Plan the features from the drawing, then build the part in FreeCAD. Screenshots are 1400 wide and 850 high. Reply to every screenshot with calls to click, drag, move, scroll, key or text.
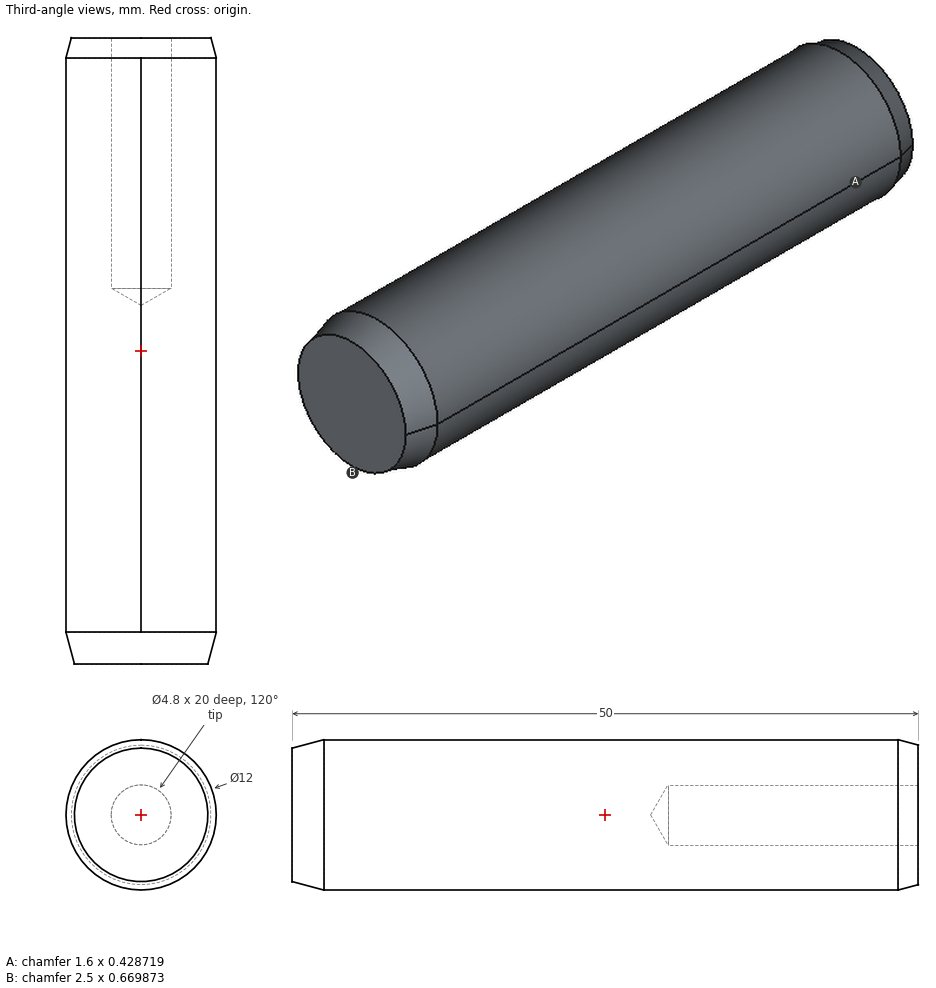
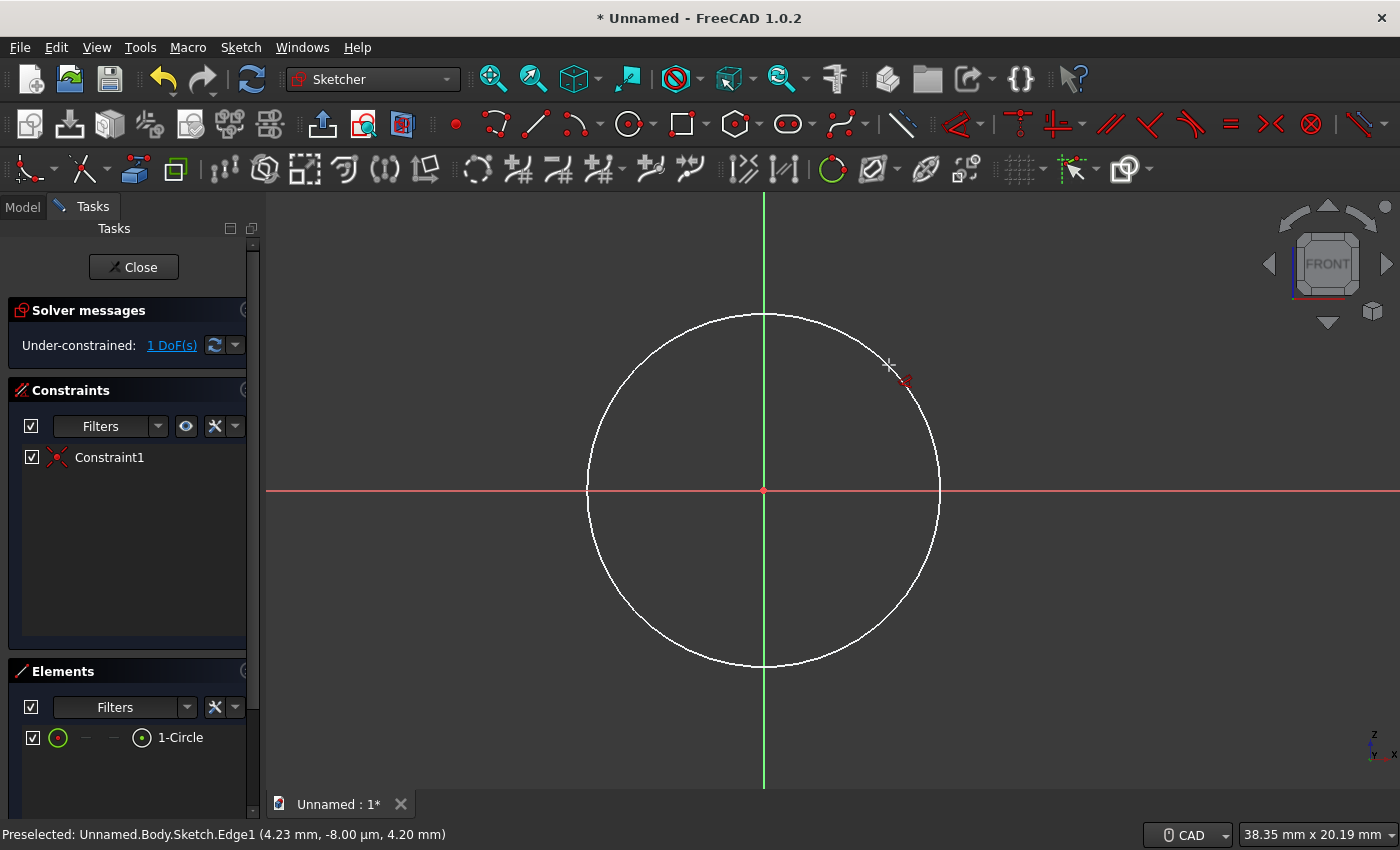
click(888, 365)
click(911, 342)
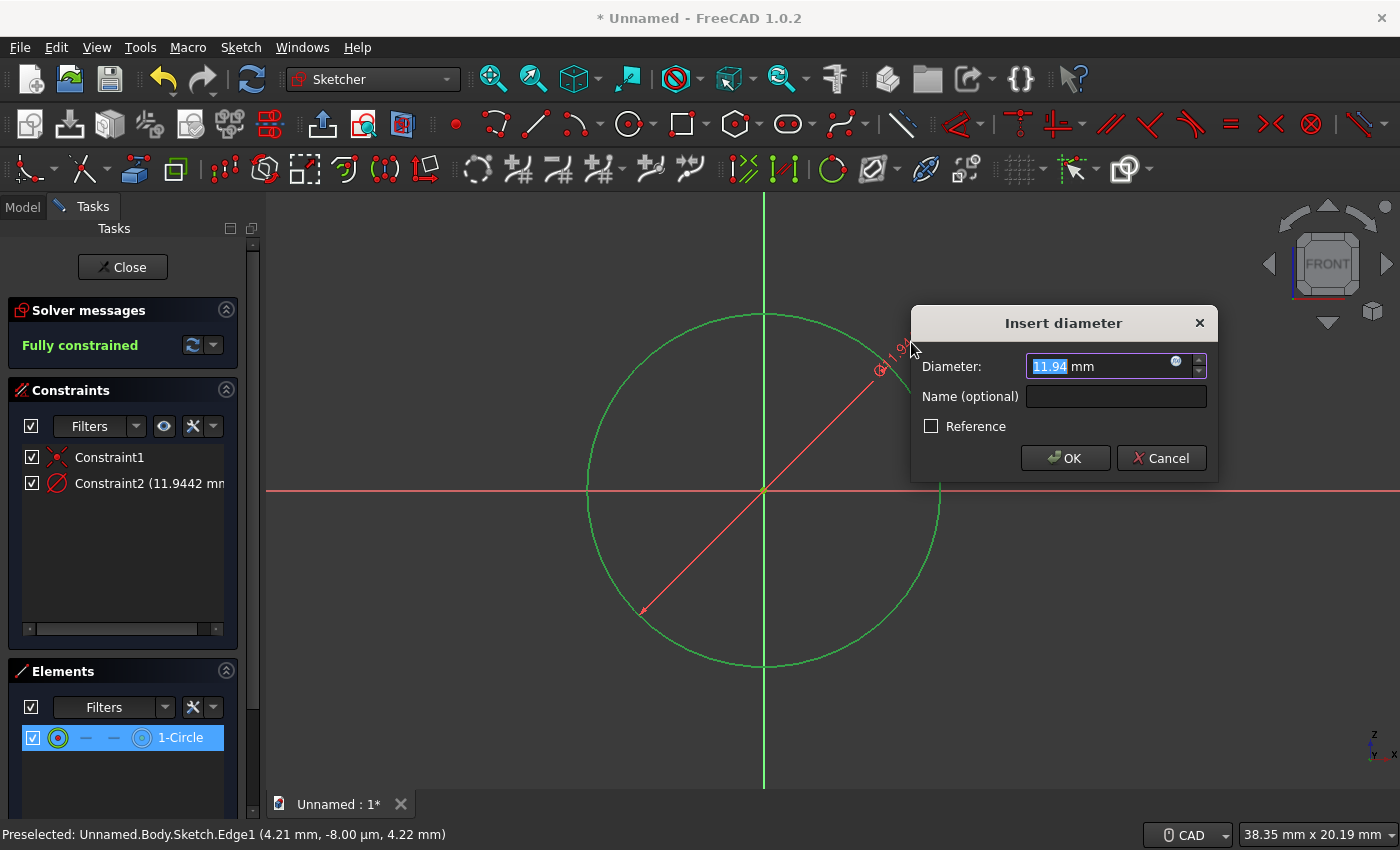
text(12)
key(Return)
key(Escape)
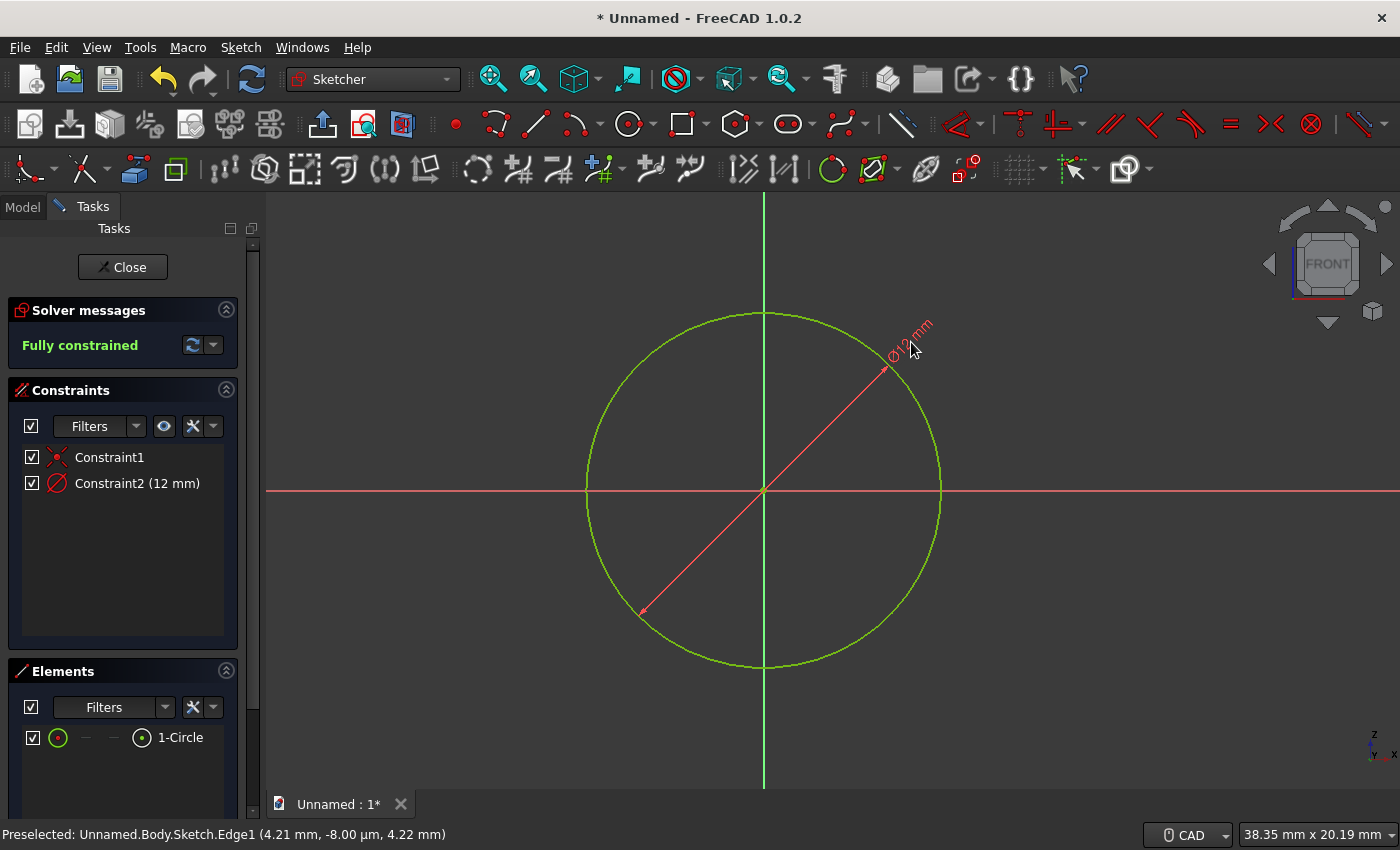
click(123, 267)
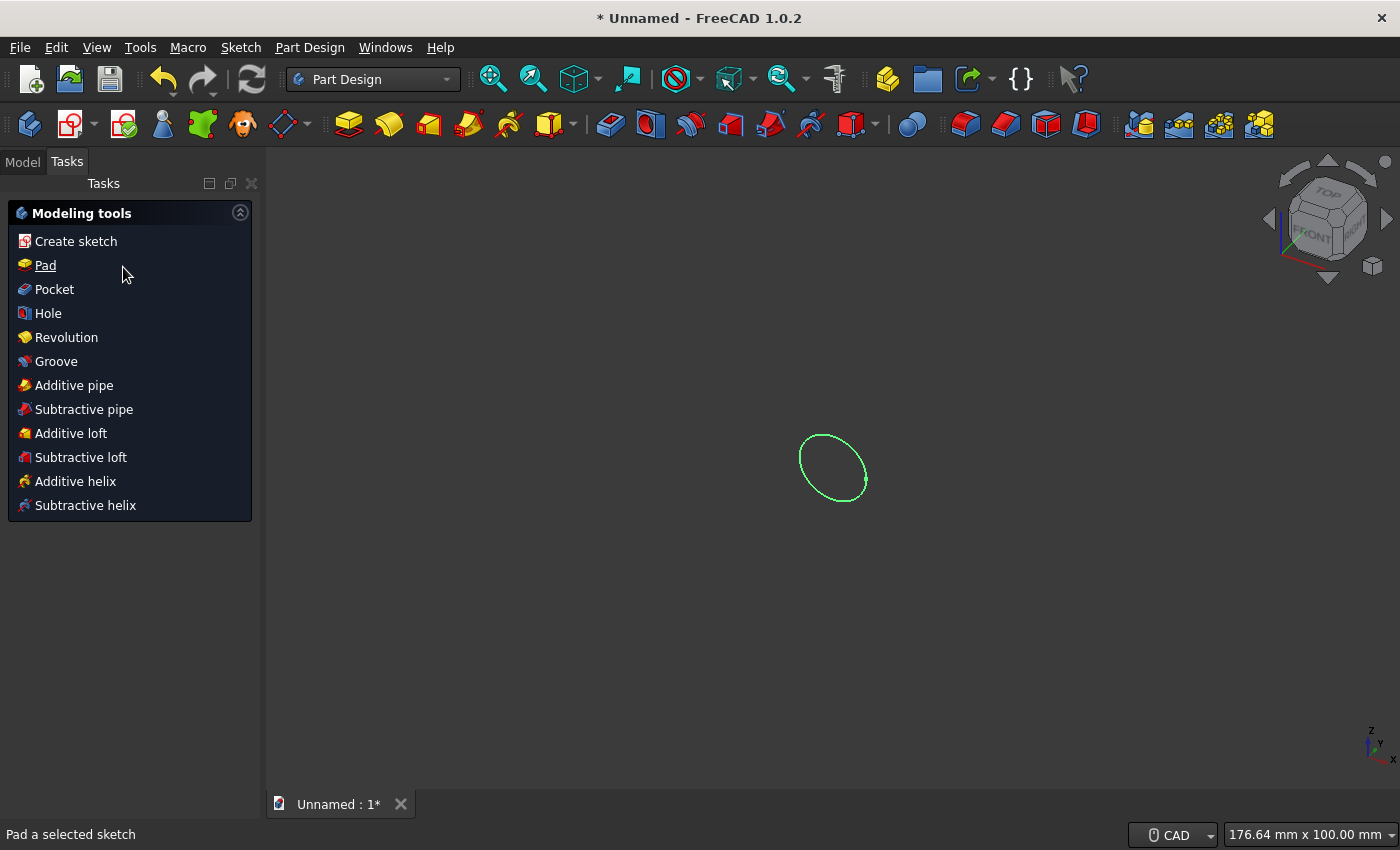
click(350, 124)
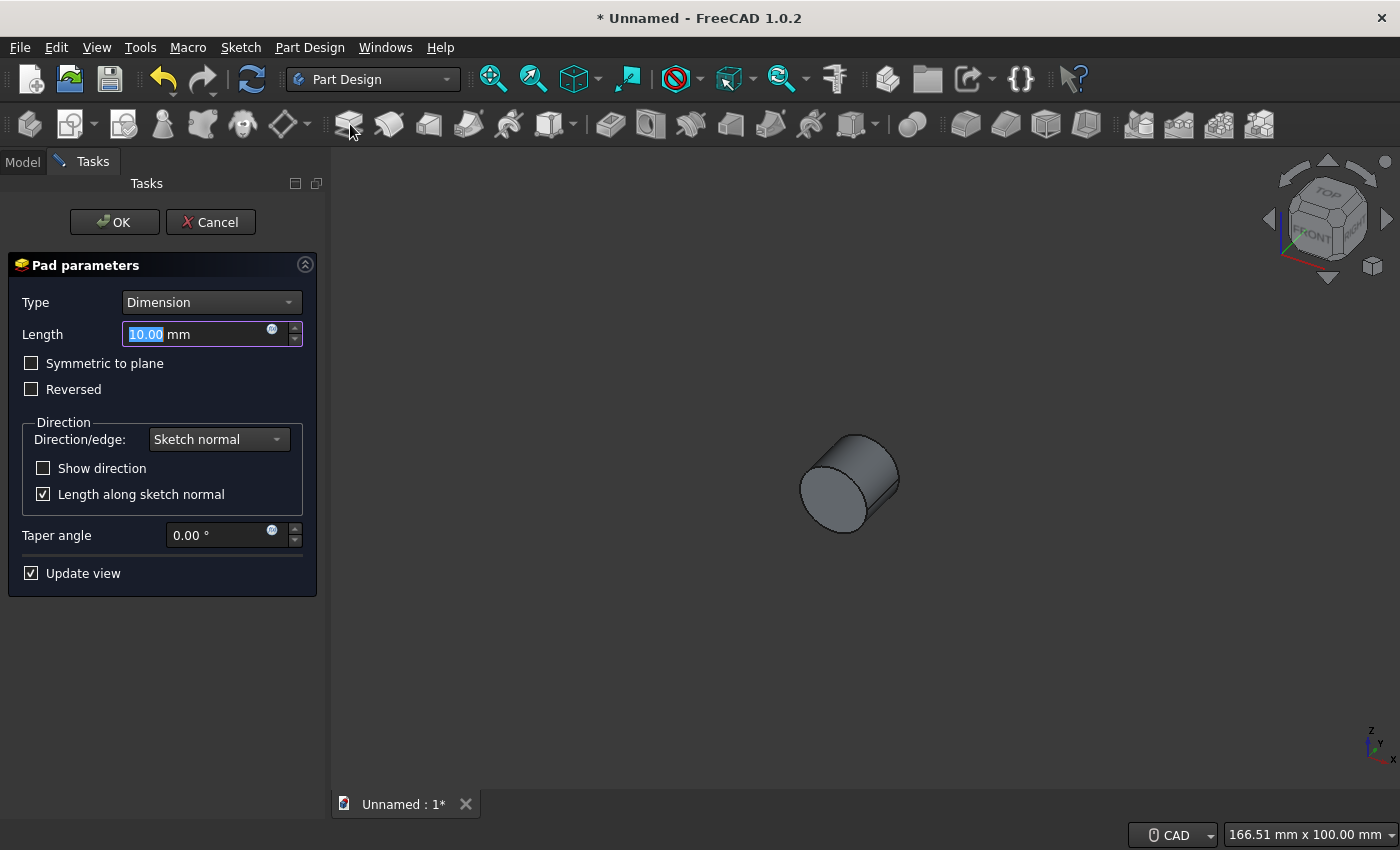
text(50)
key(Tab)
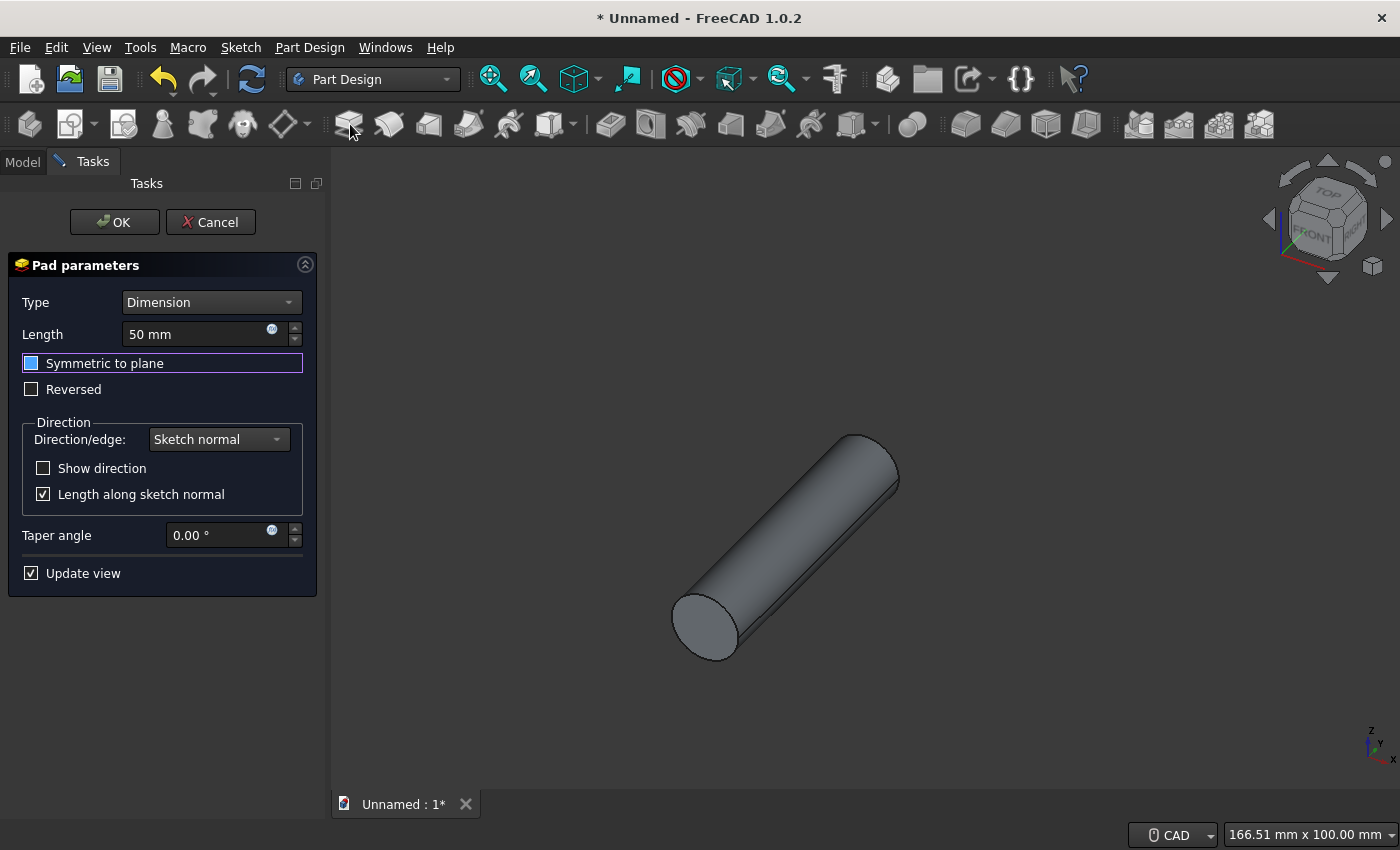
click(30, 363)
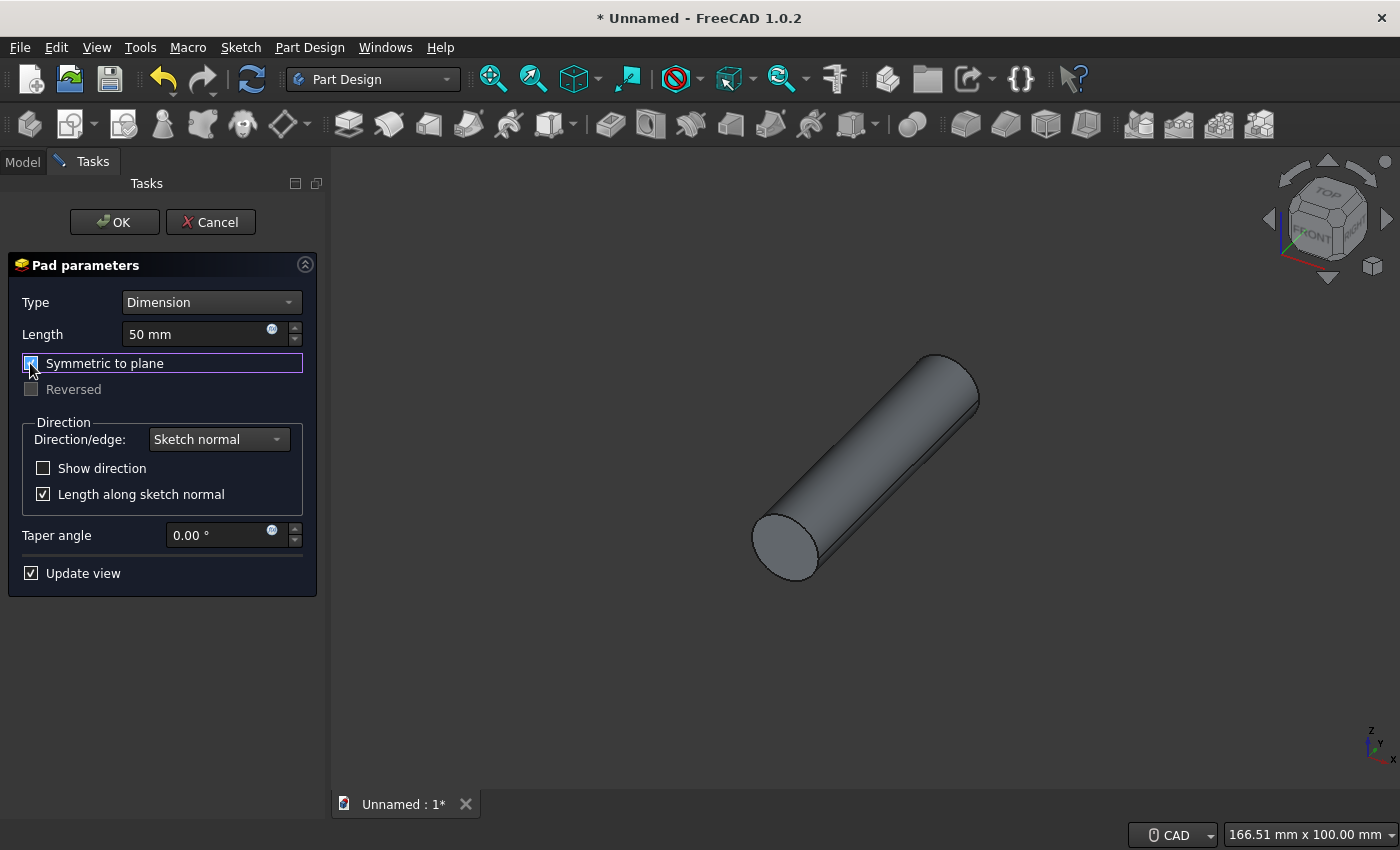
click(115, 222)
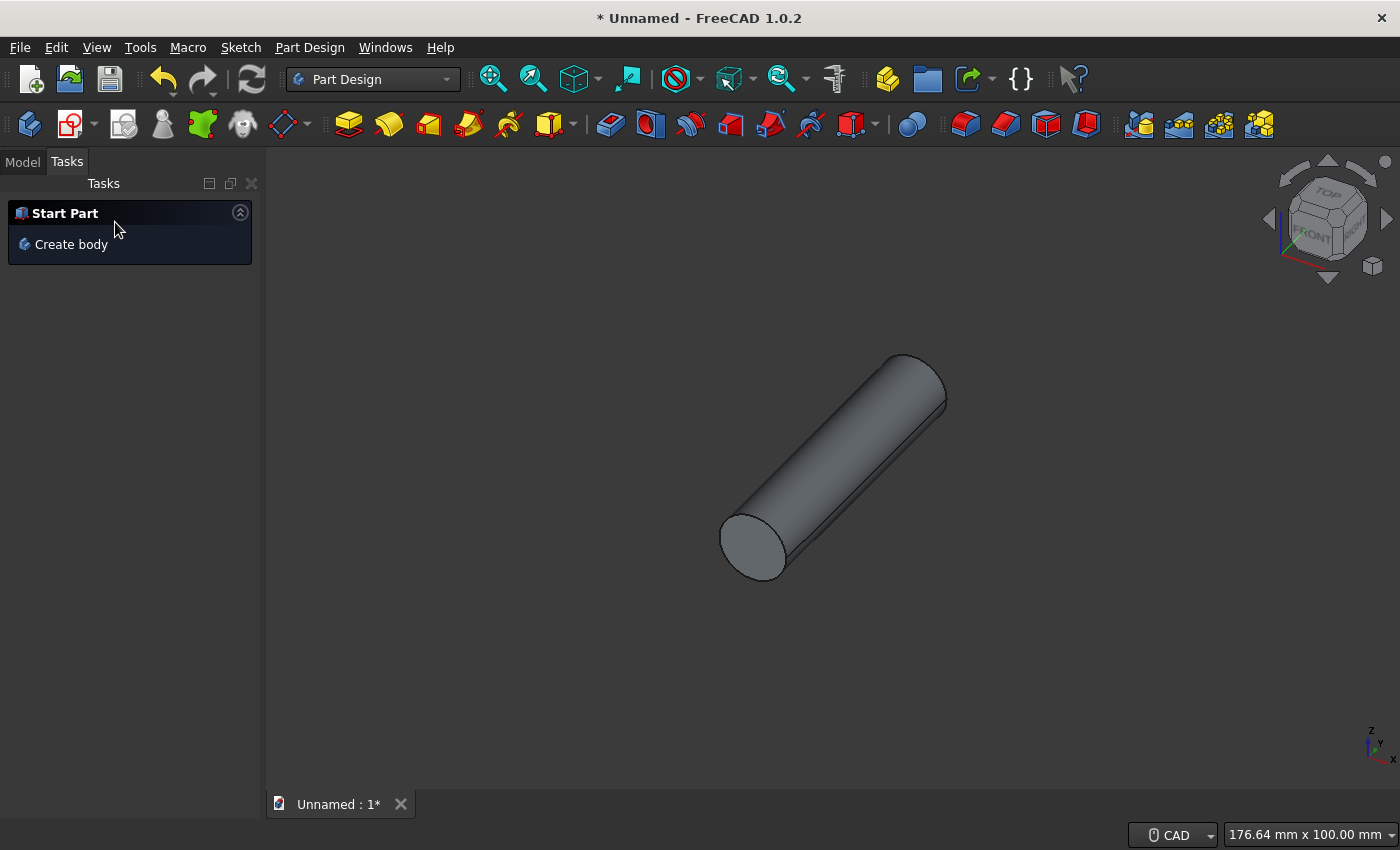
click(494, 80)